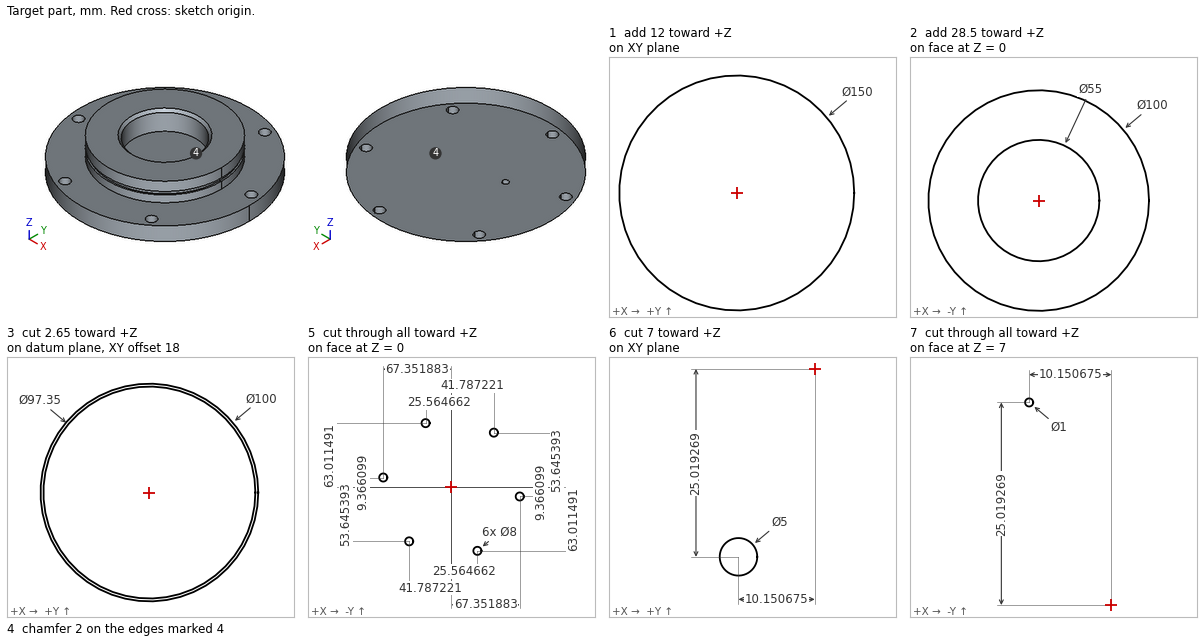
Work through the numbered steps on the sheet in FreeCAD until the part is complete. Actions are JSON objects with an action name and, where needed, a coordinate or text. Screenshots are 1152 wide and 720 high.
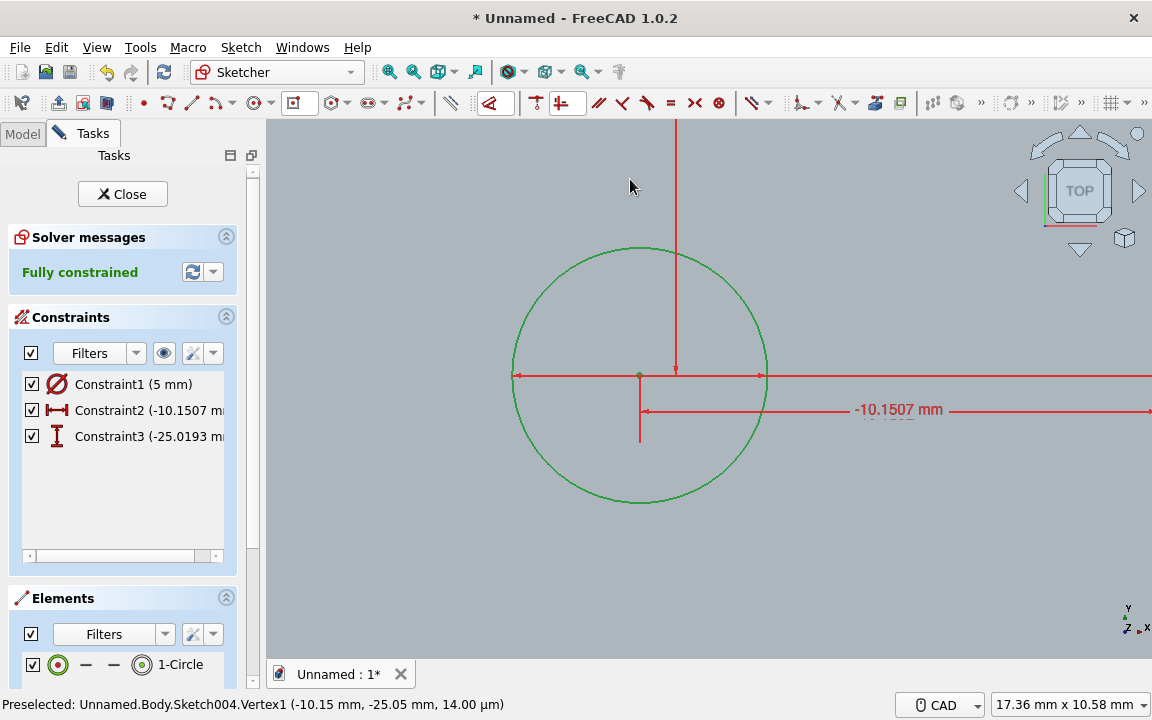
{"action": "left_click", "coordinate": [123, 194]}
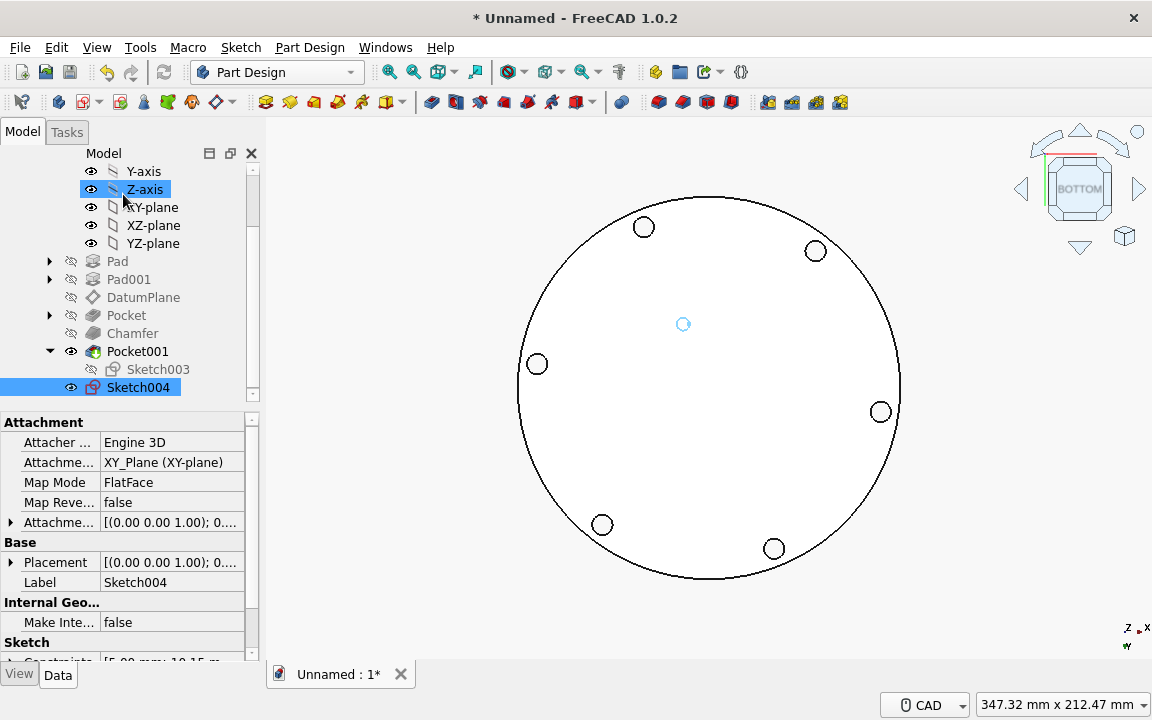
{"action": "left_click", "coordinate": [432, 102]}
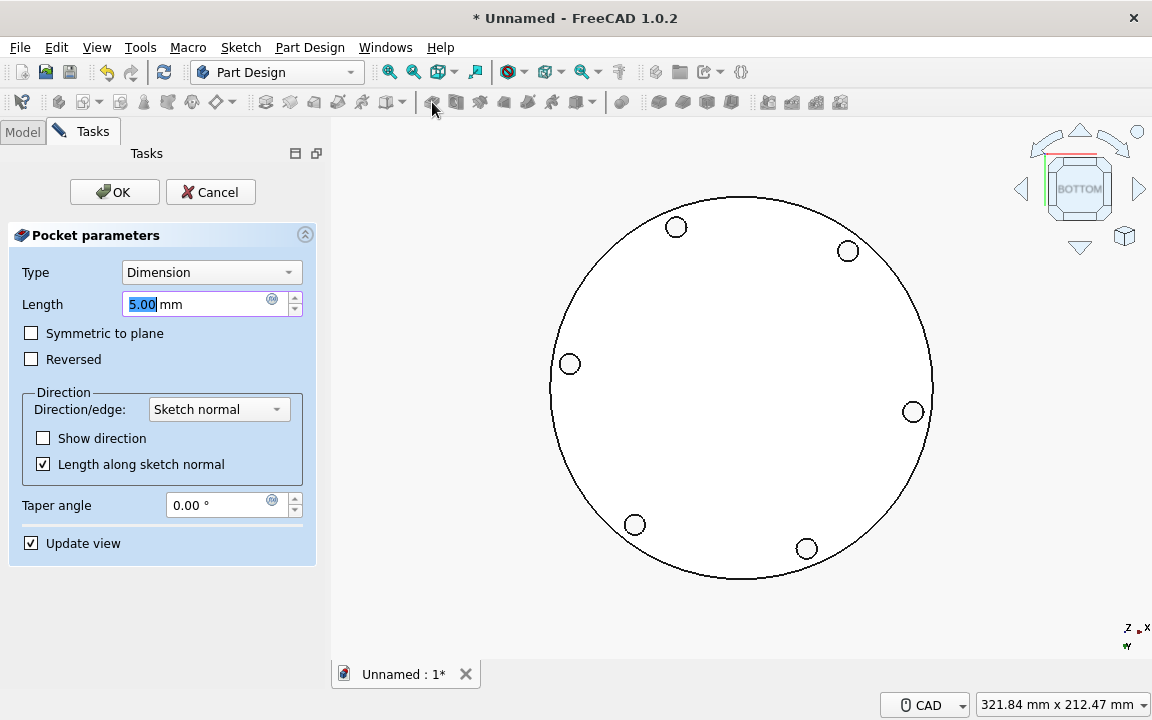
{"action": "type", "text": "7"}
{"action": "key", "text": "Tab"}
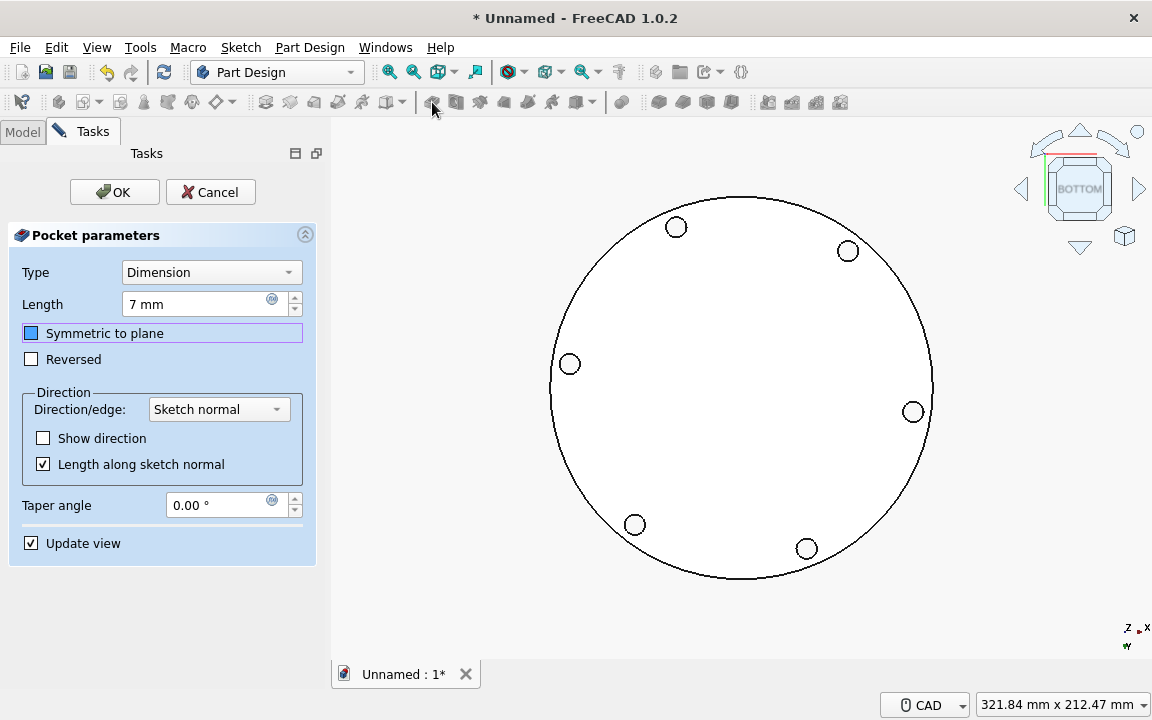
{"action": "left_click", "coordinate": [30, 359]}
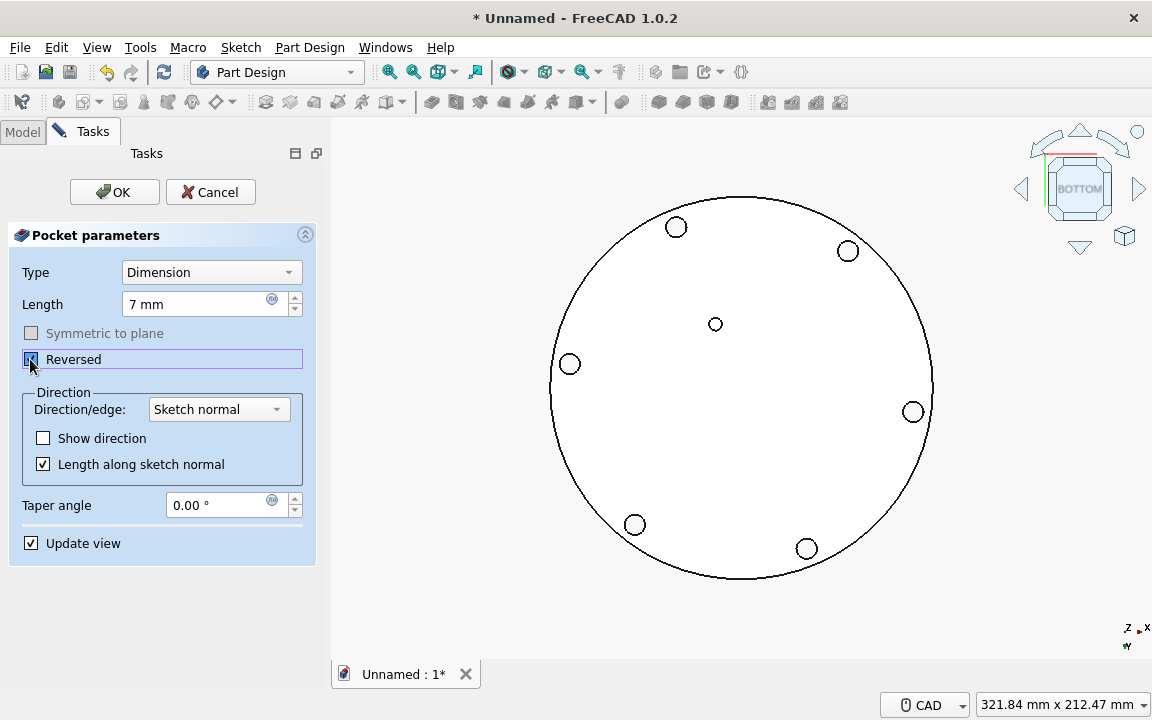
{"action": "left_click", "coordinate": [115, 192]}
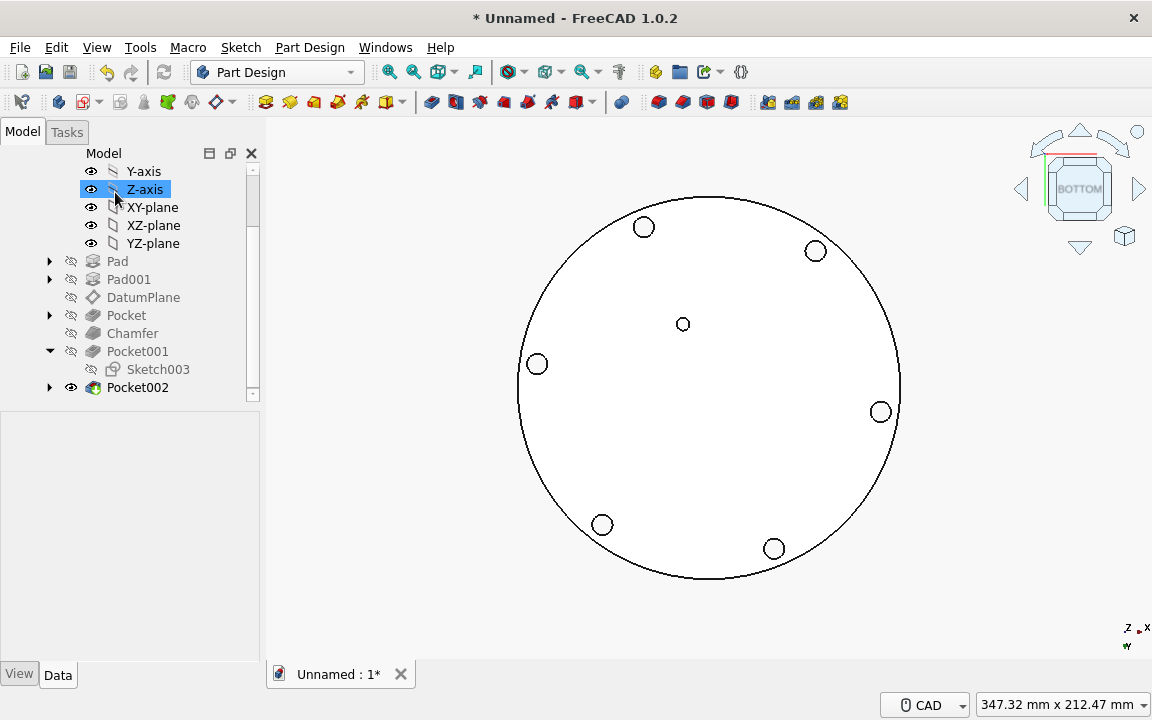
{"action": "scroll", "coordinate": [683, 323], "scroll_direction": "up", "scroll_amount": 4}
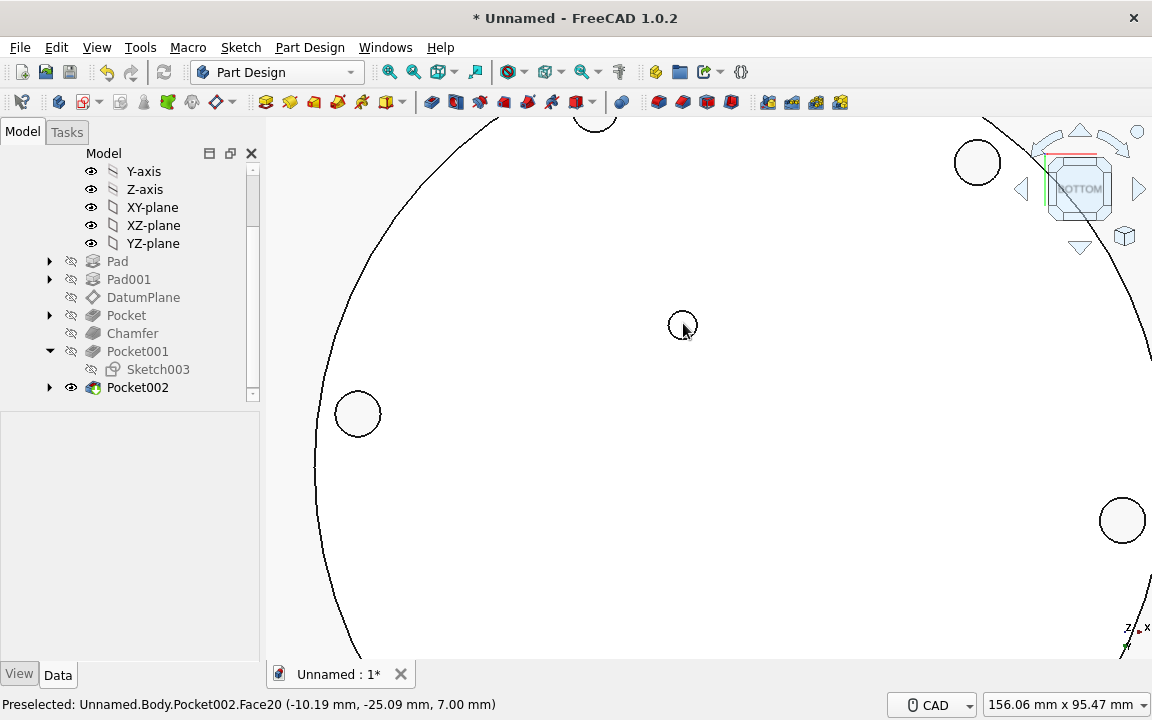
{"action": "left_click", "coordinate": [683, 324]}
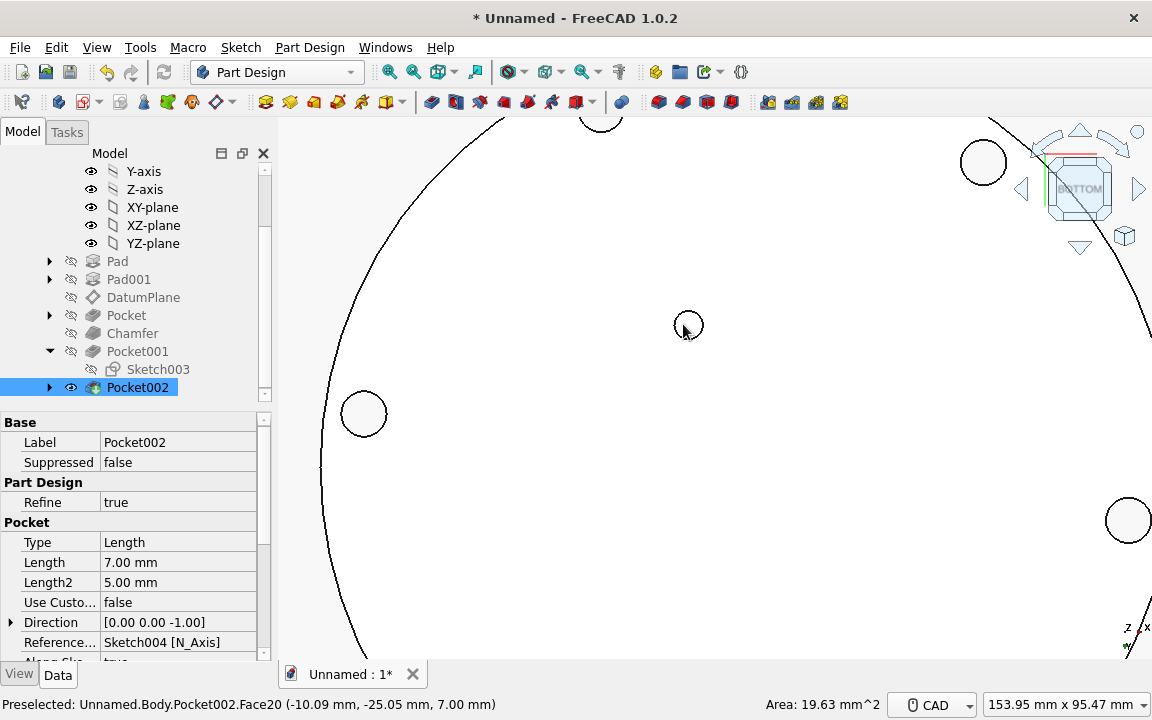
{"action": "left_click", "coordinate": [84, 102]}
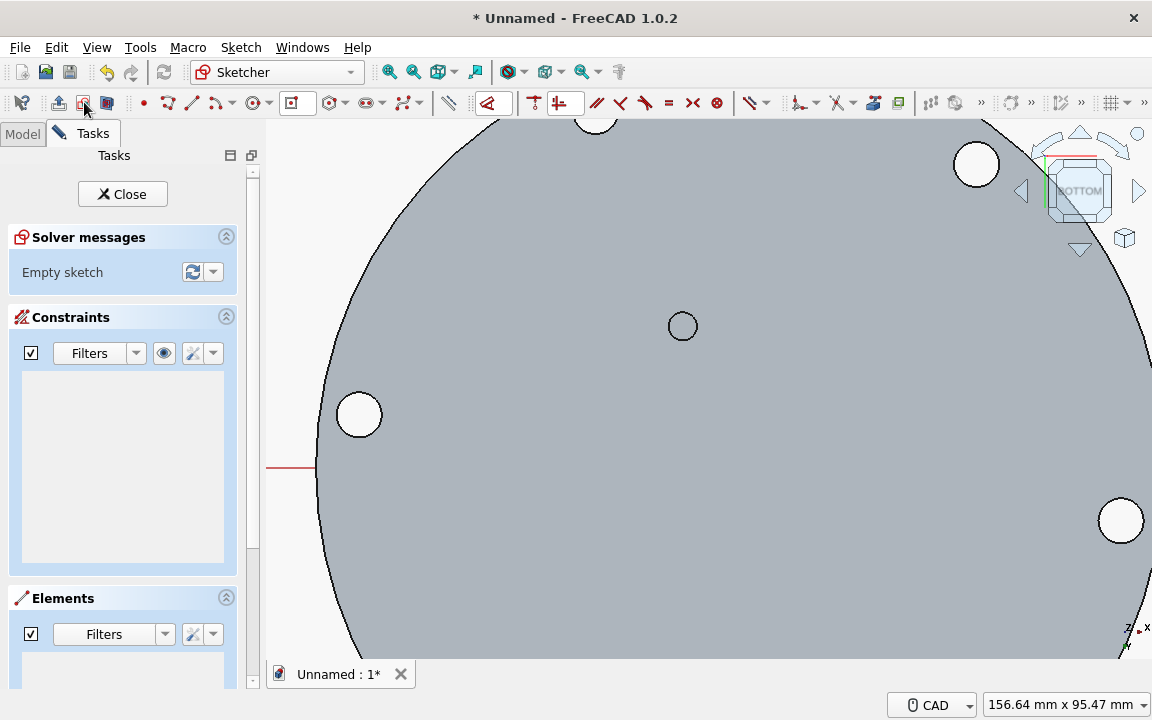
{"action": "scroll", "coordinate": [685, 323], "scroll_direction": "up", "scroll_amount": 15}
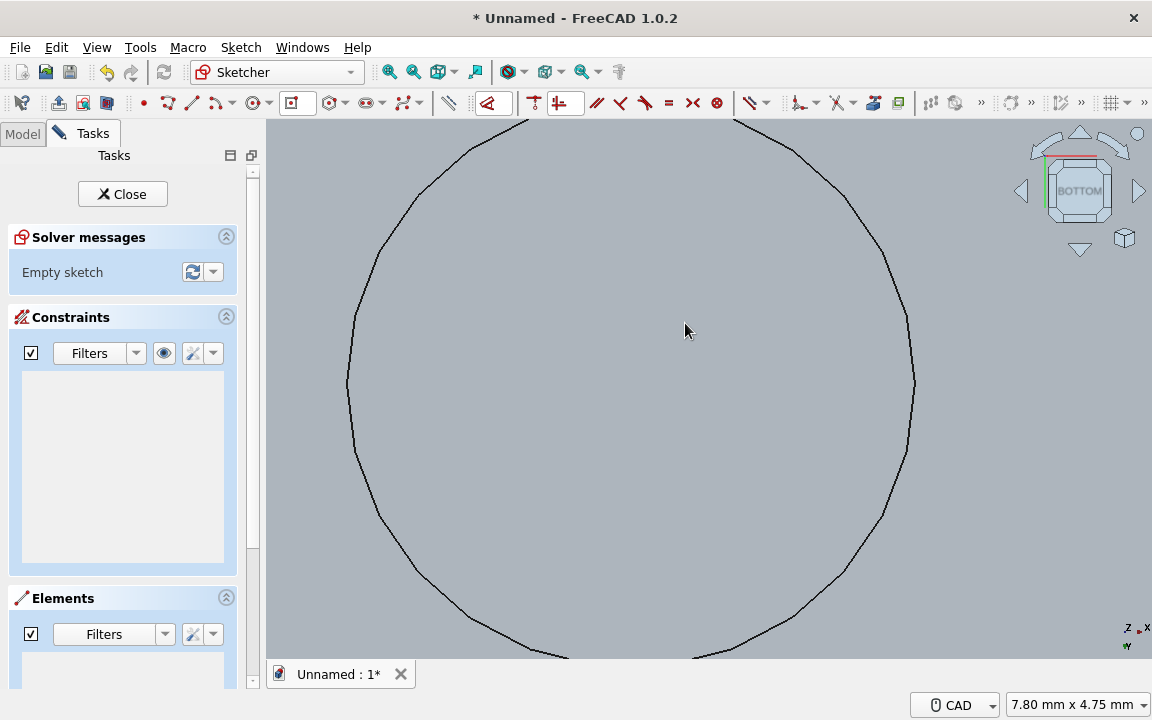
{"action": "scroll", "coordinate": [627, 382], "scroll_direction": "up", "scroll_amount": 6}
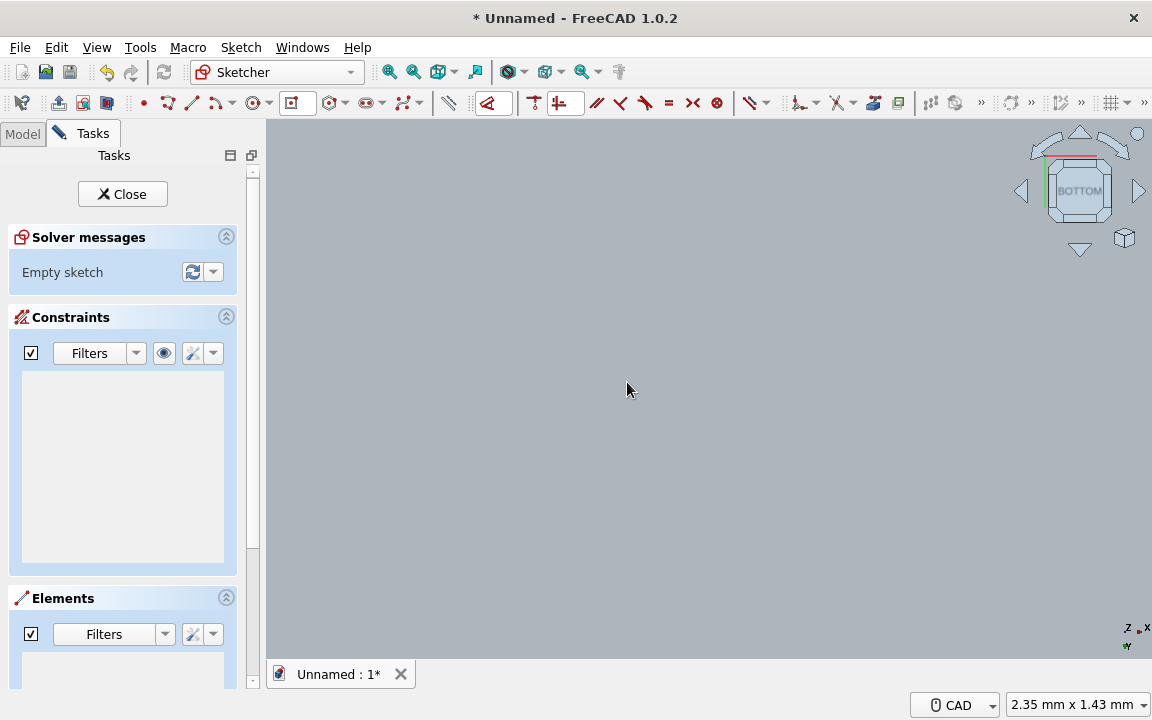
{"action": "left_click", "coordinate": [254, 104]}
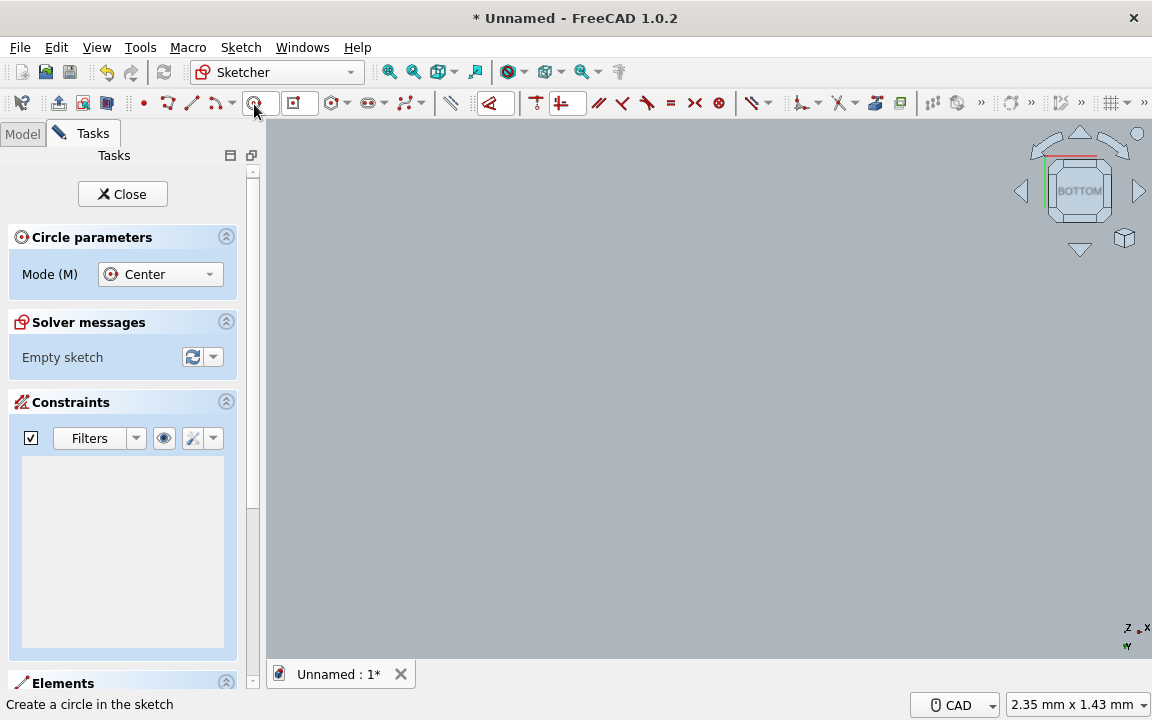
{"action": "left_click", "coordinate": [639, 387]}
{"action": "mouse_move", "coordinate": [772, 253]}